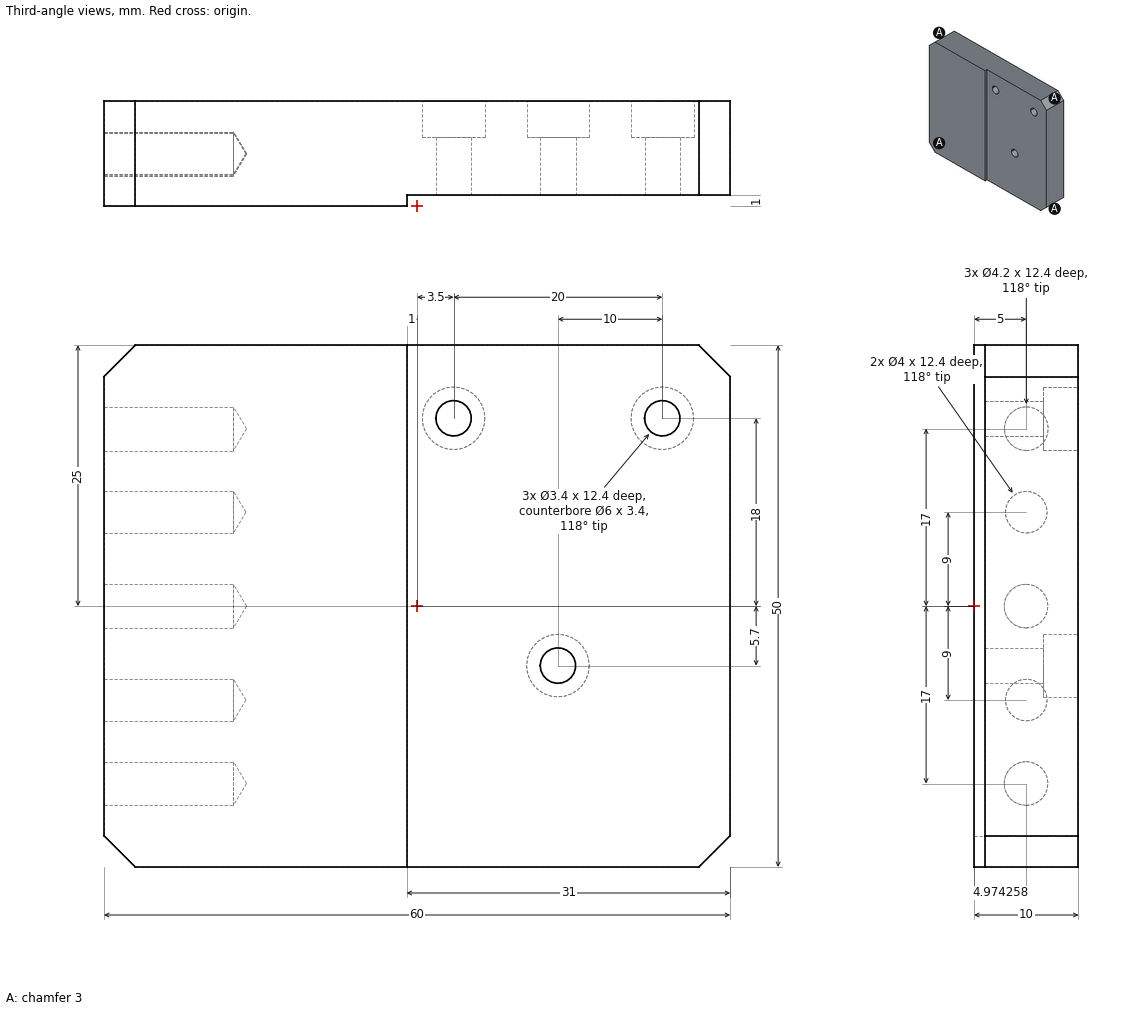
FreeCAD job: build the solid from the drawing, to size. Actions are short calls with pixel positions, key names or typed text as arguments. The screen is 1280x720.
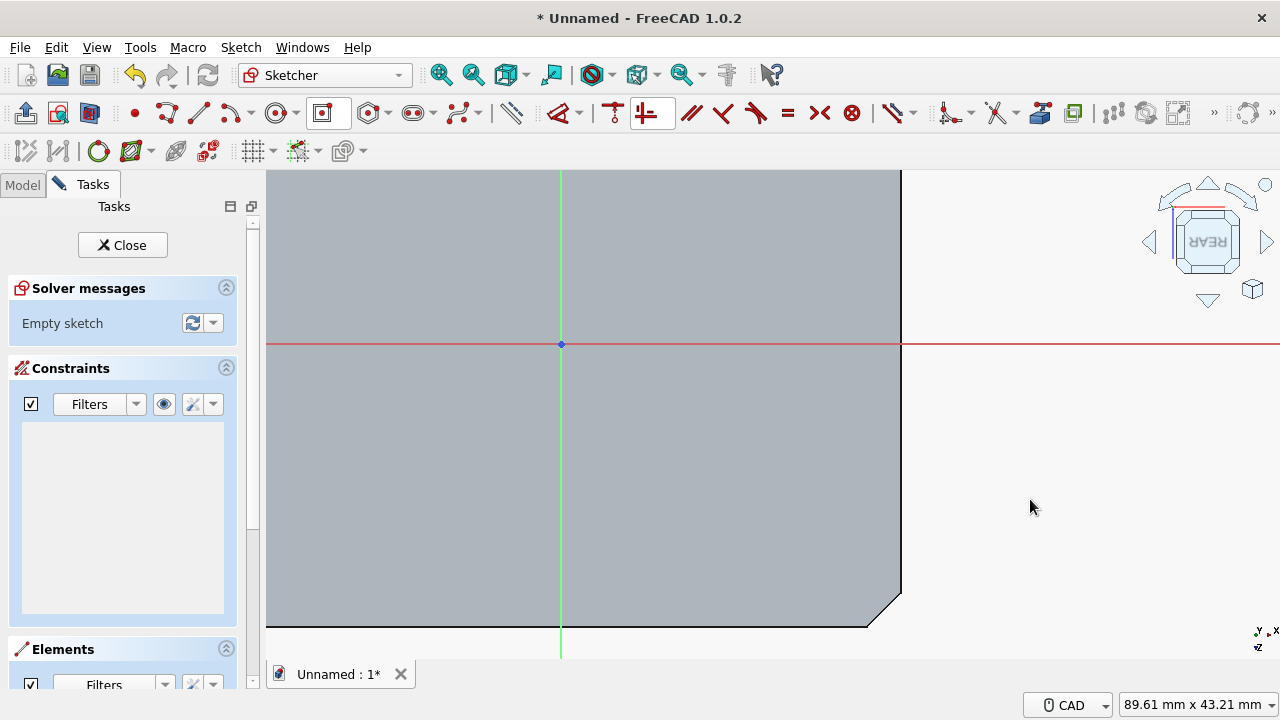
click(276, 114)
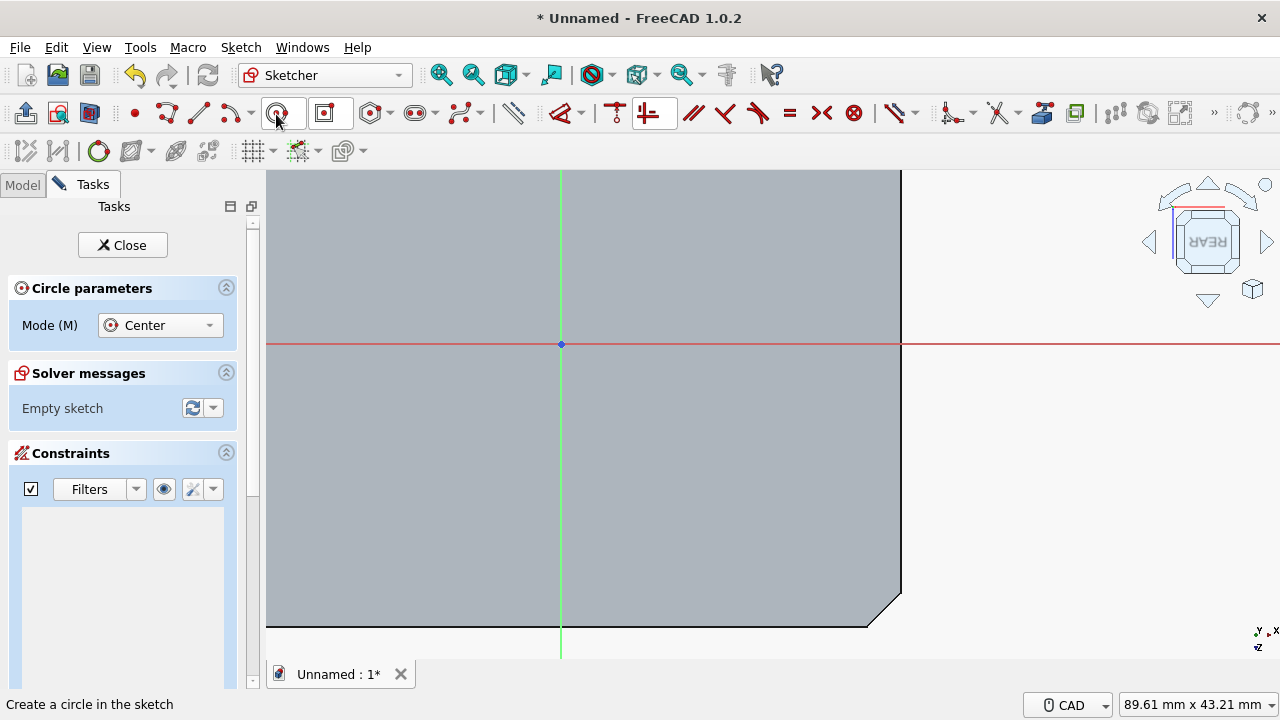
click(827, 548)
move(841, 535)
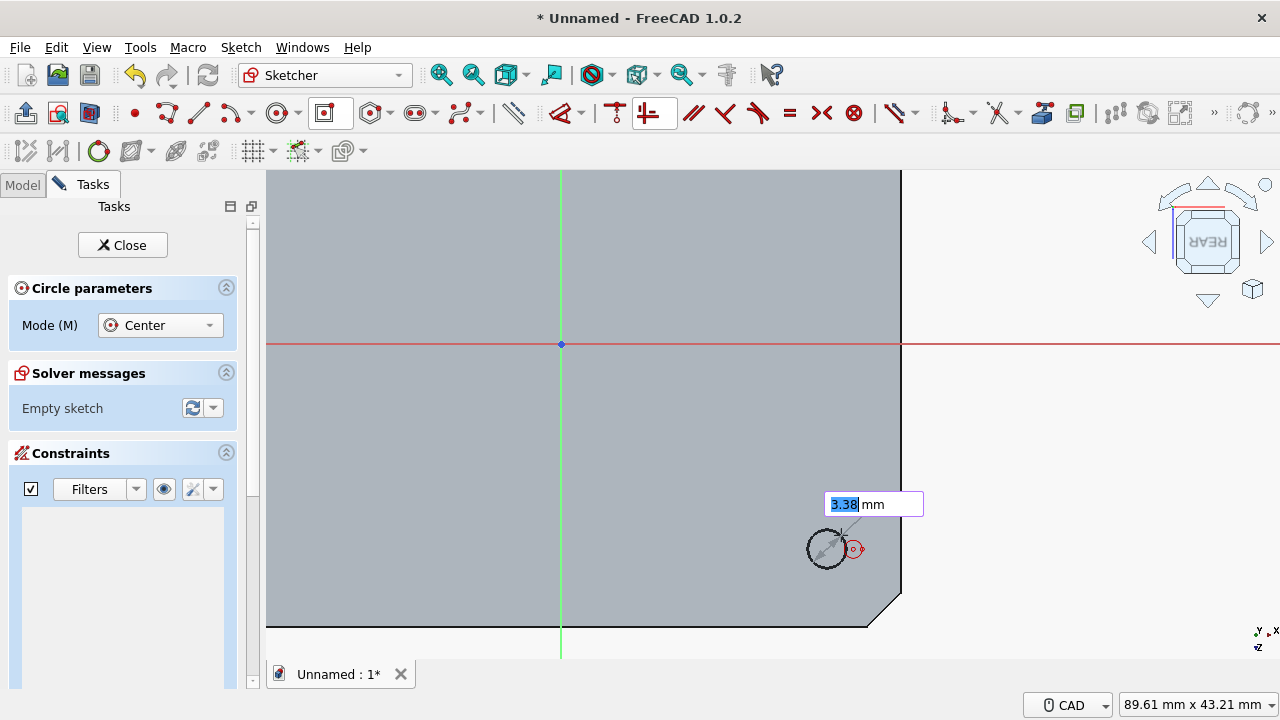
text(3.4)
key(Return)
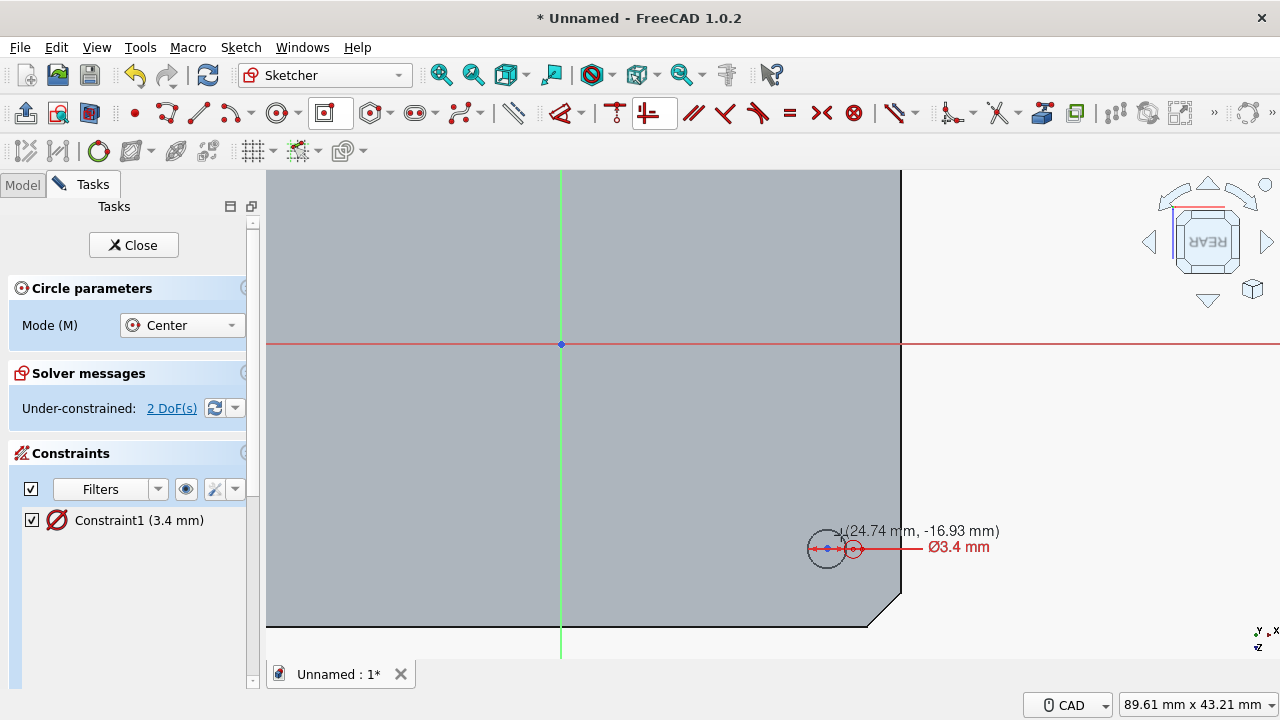
click(601, 548)
move(614, 535)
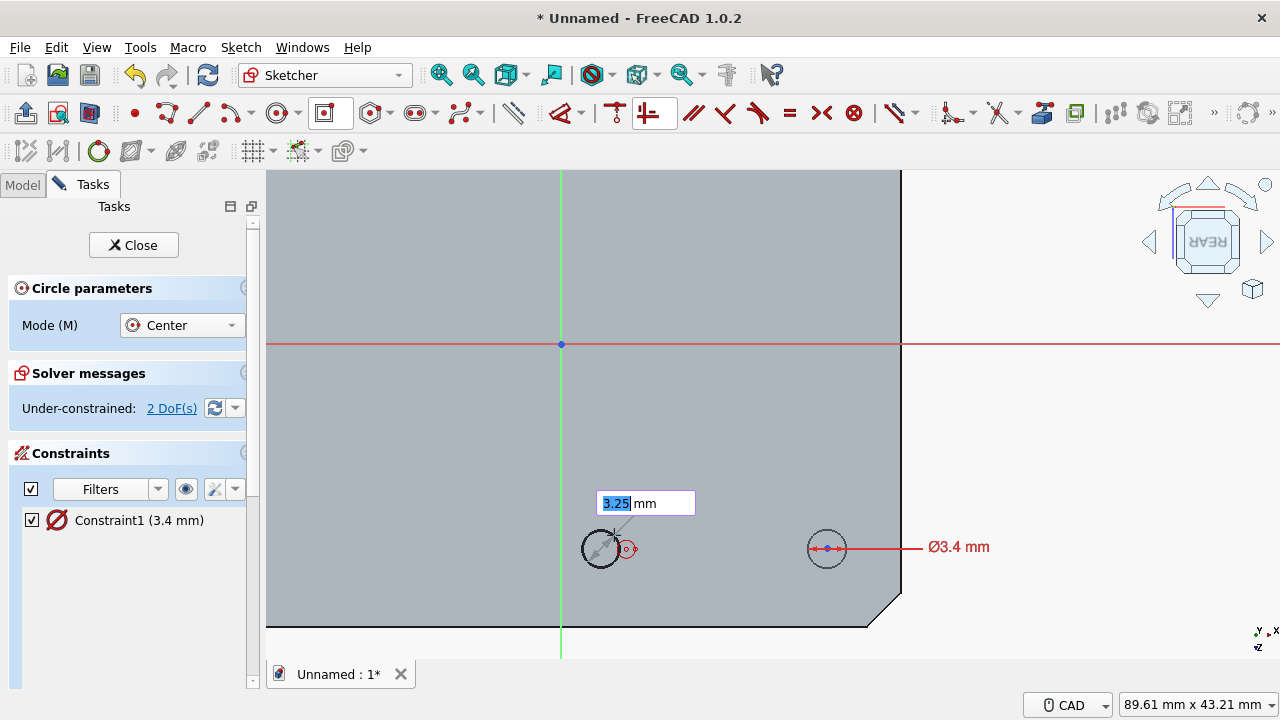
text(3.4)
key(Return)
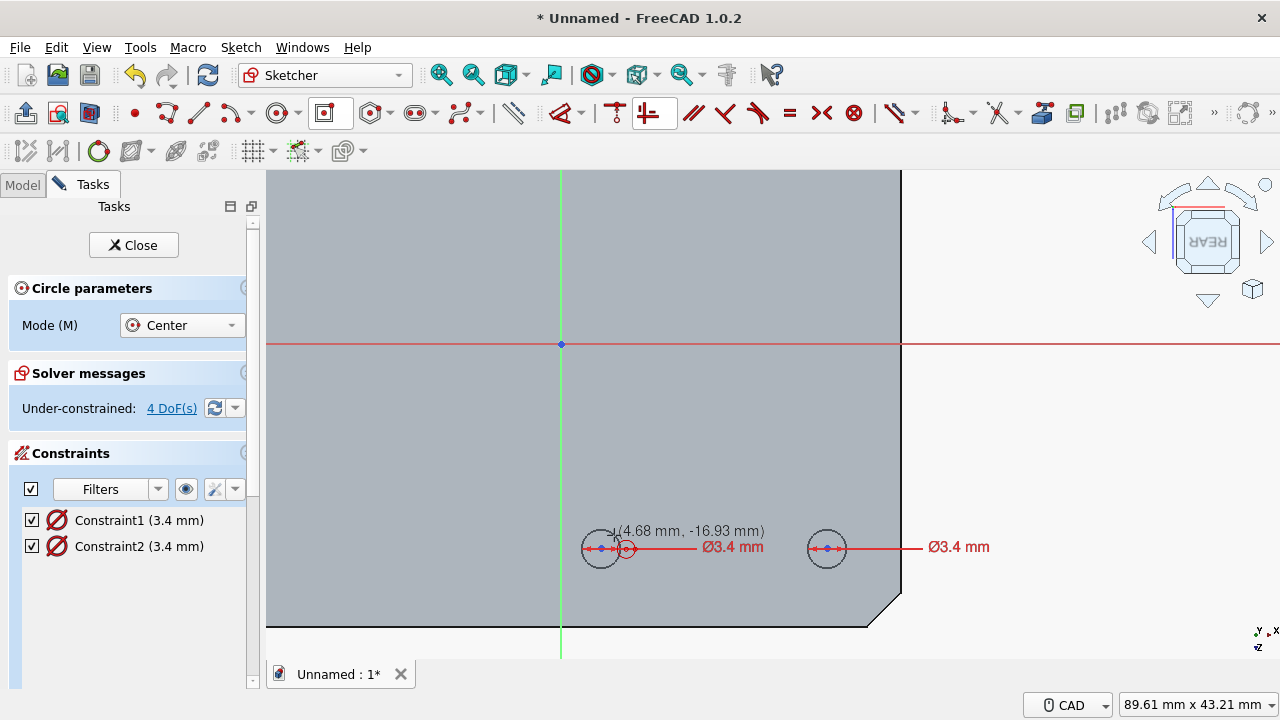
click(714, 280)
move(727, 266)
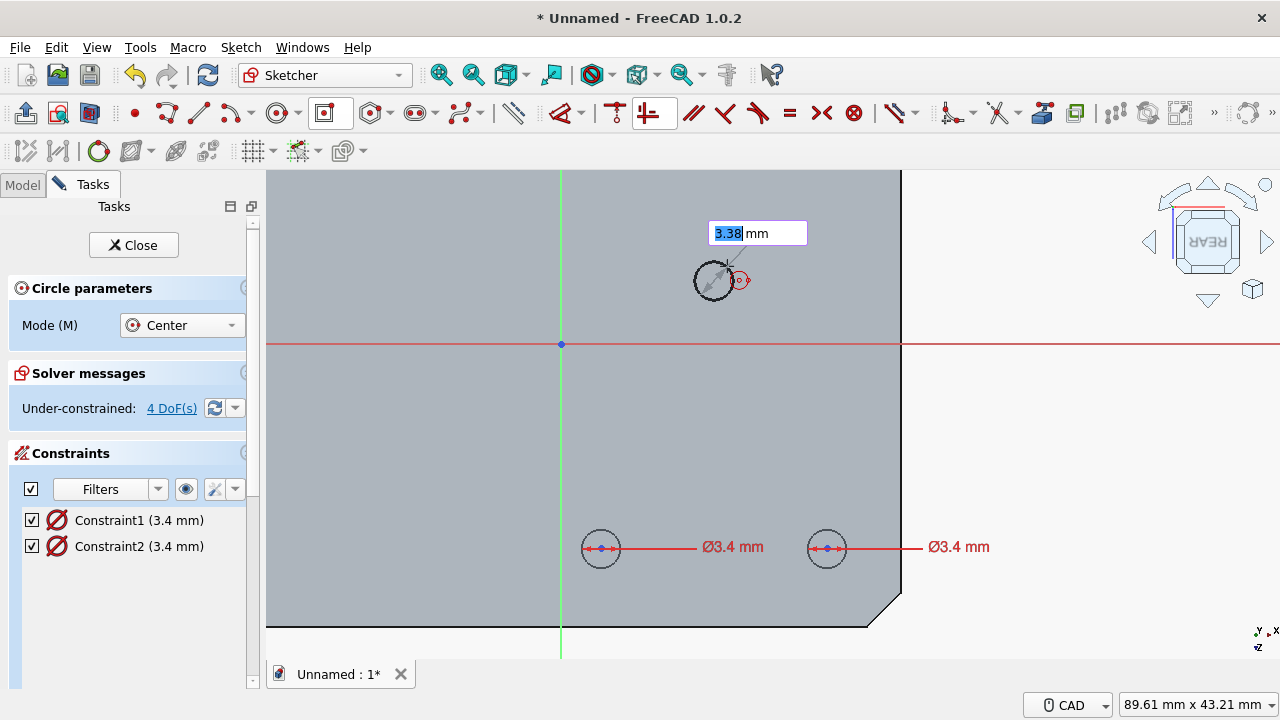
text(3.4)
key(Return)
key(Escape)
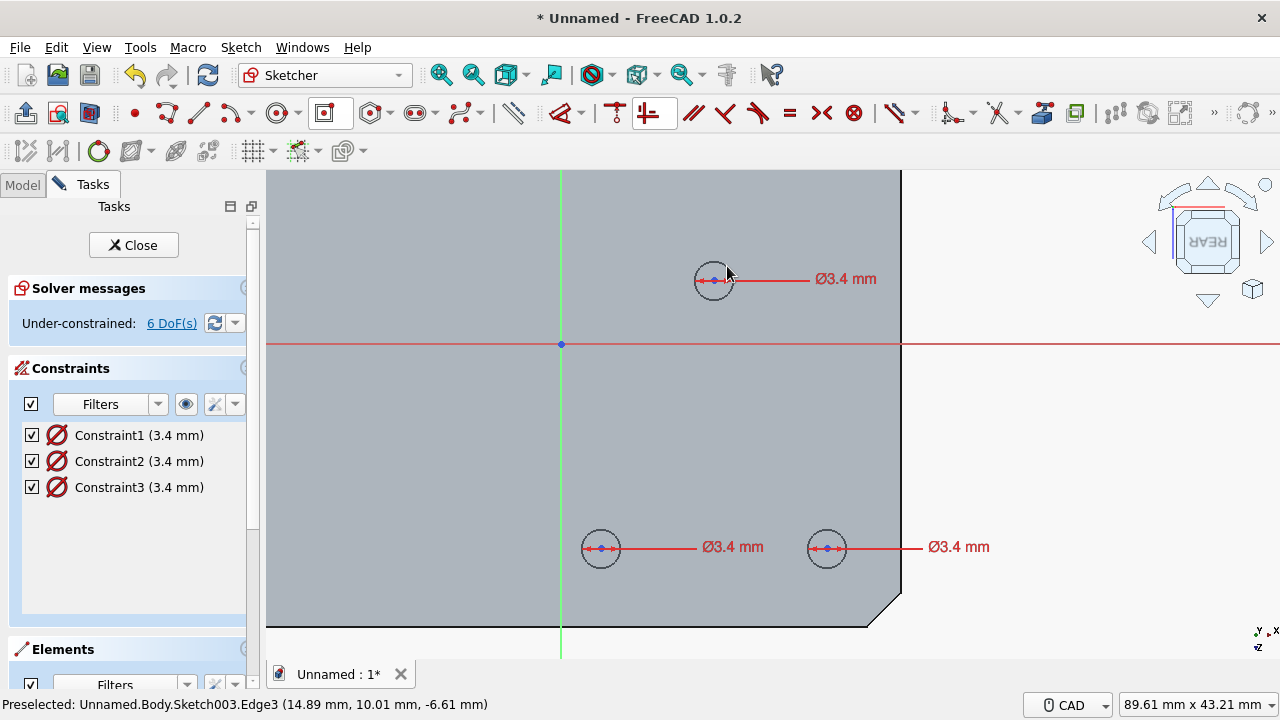
click(827, 549)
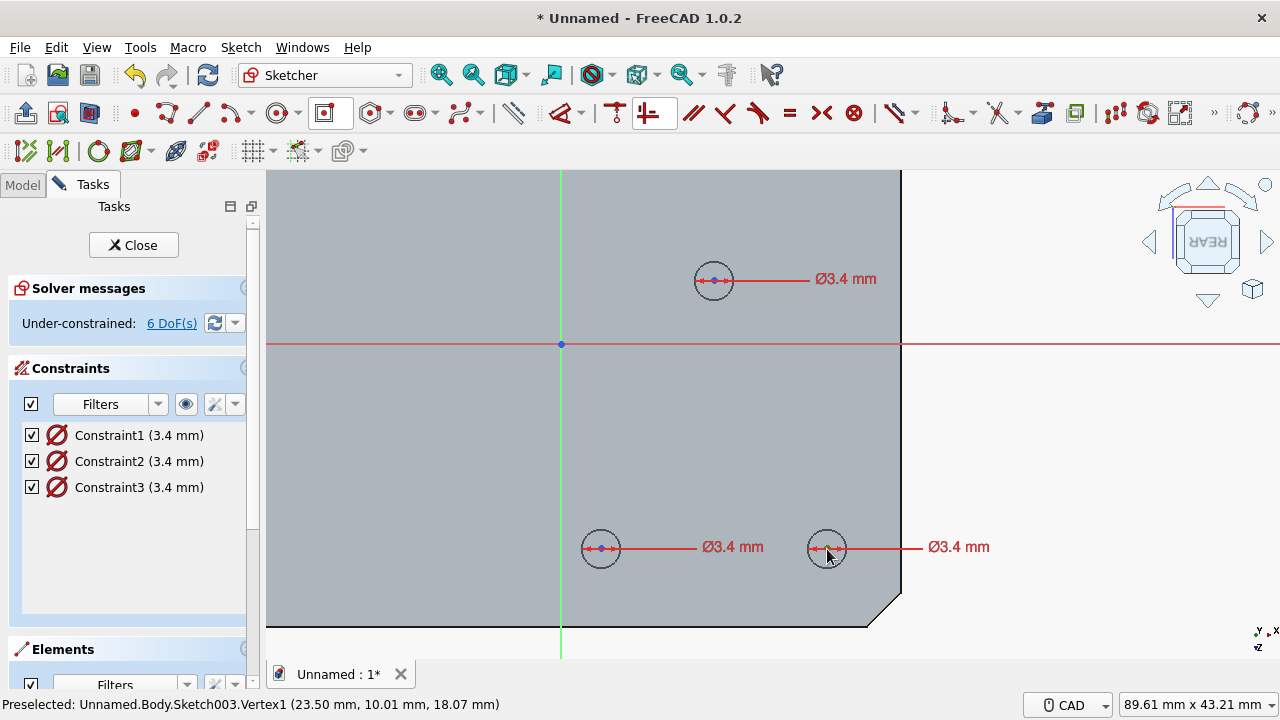
click(601, 549)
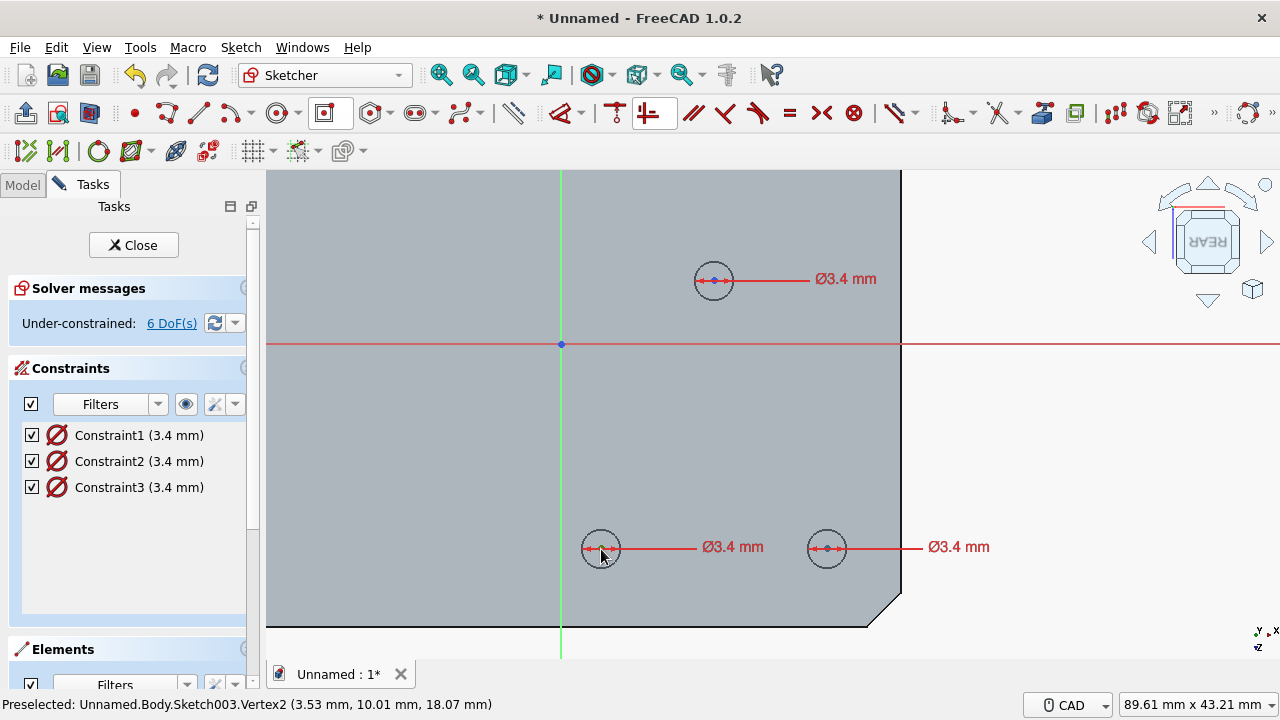
key(h)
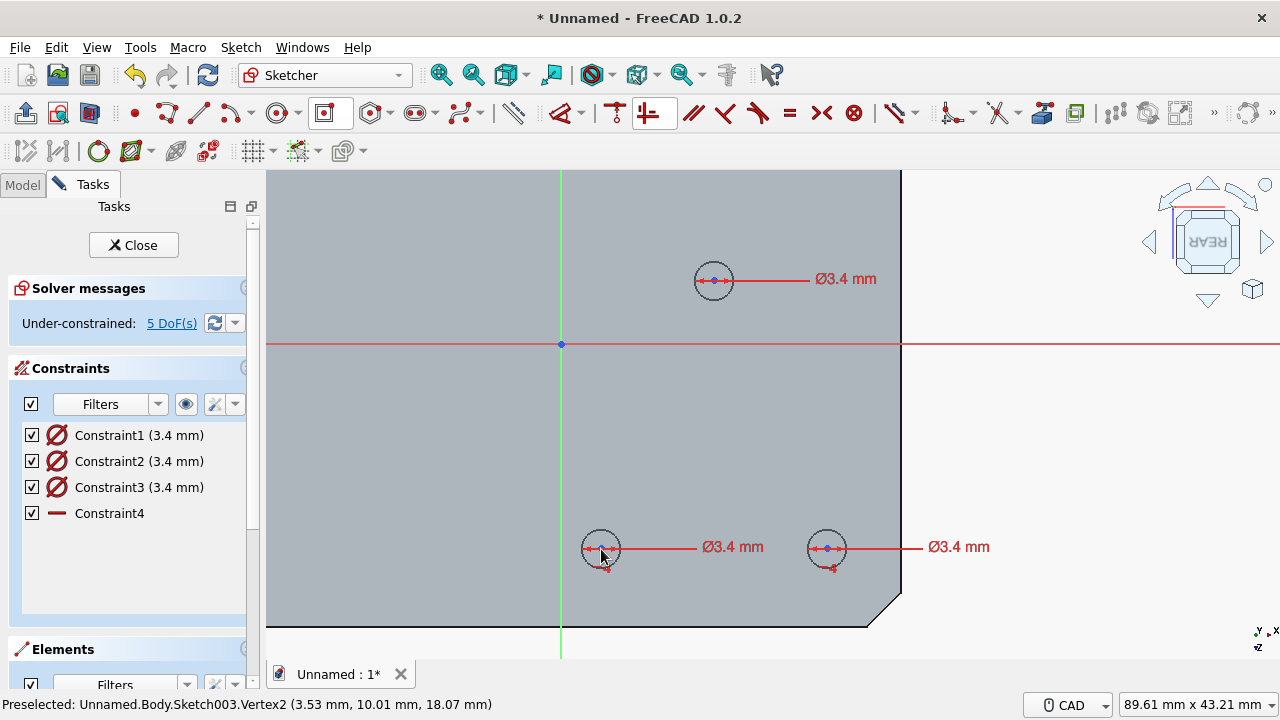
click(560, 114)